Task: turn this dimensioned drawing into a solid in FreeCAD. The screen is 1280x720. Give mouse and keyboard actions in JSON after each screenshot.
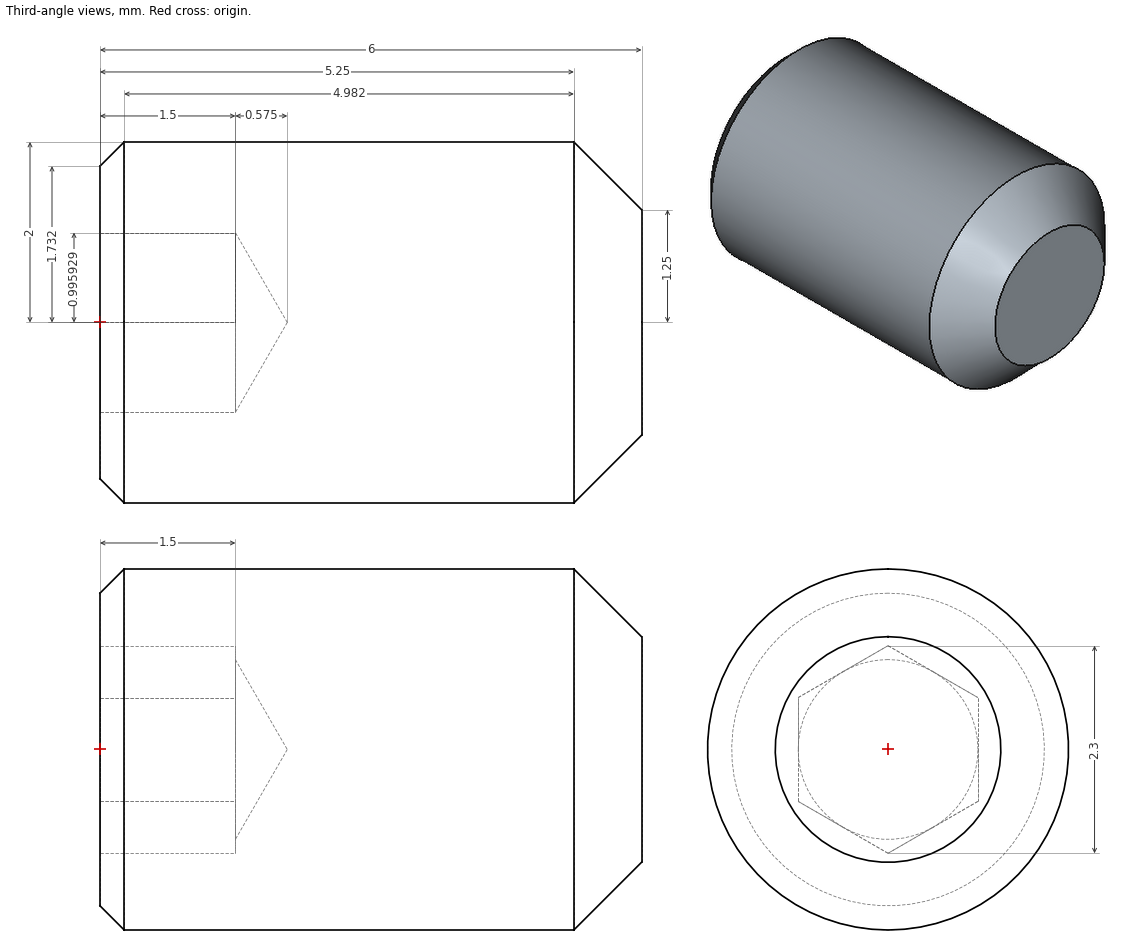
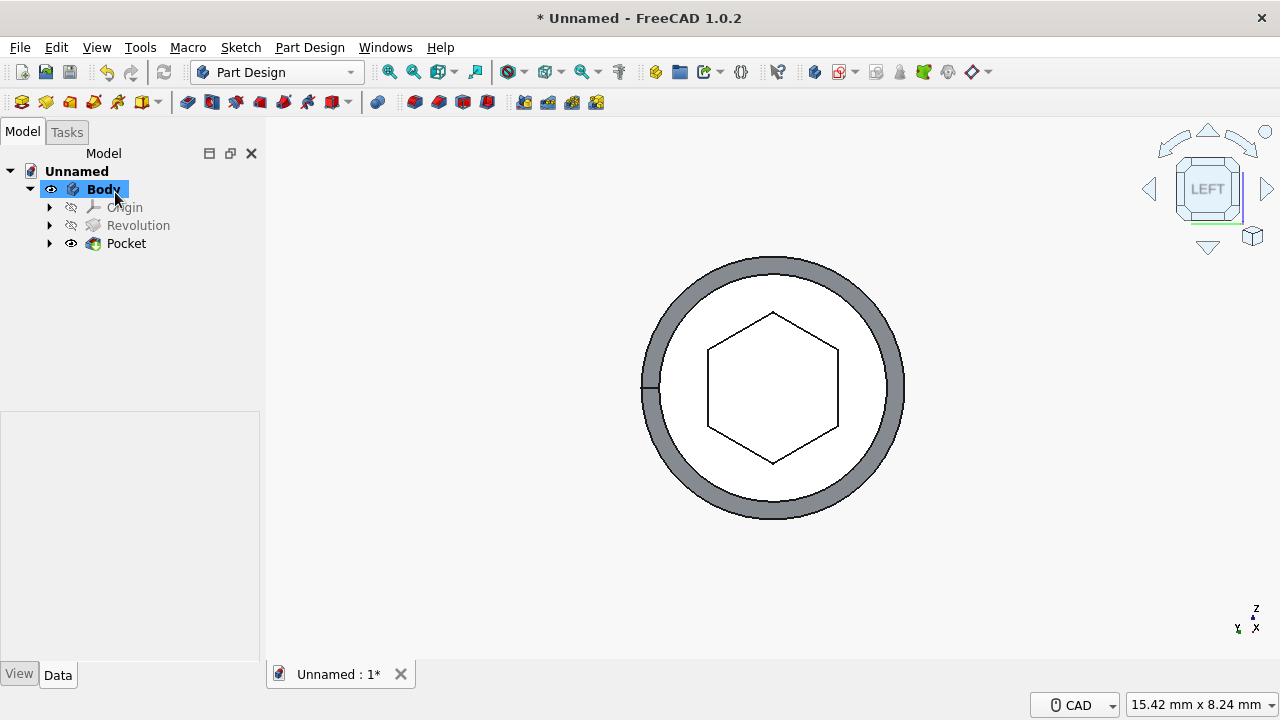
{"action": "left_click", "coordinate": [840, 72]}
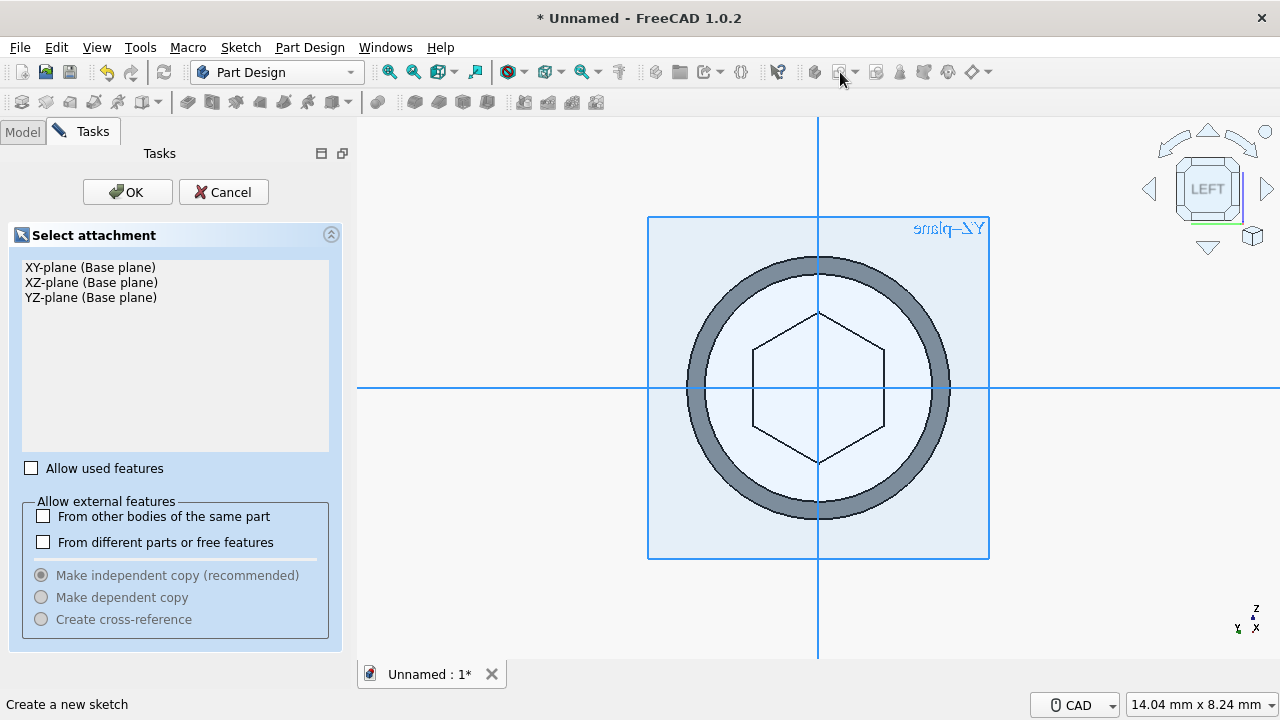
{"action": "left_click", "coordinate": [82, 268]}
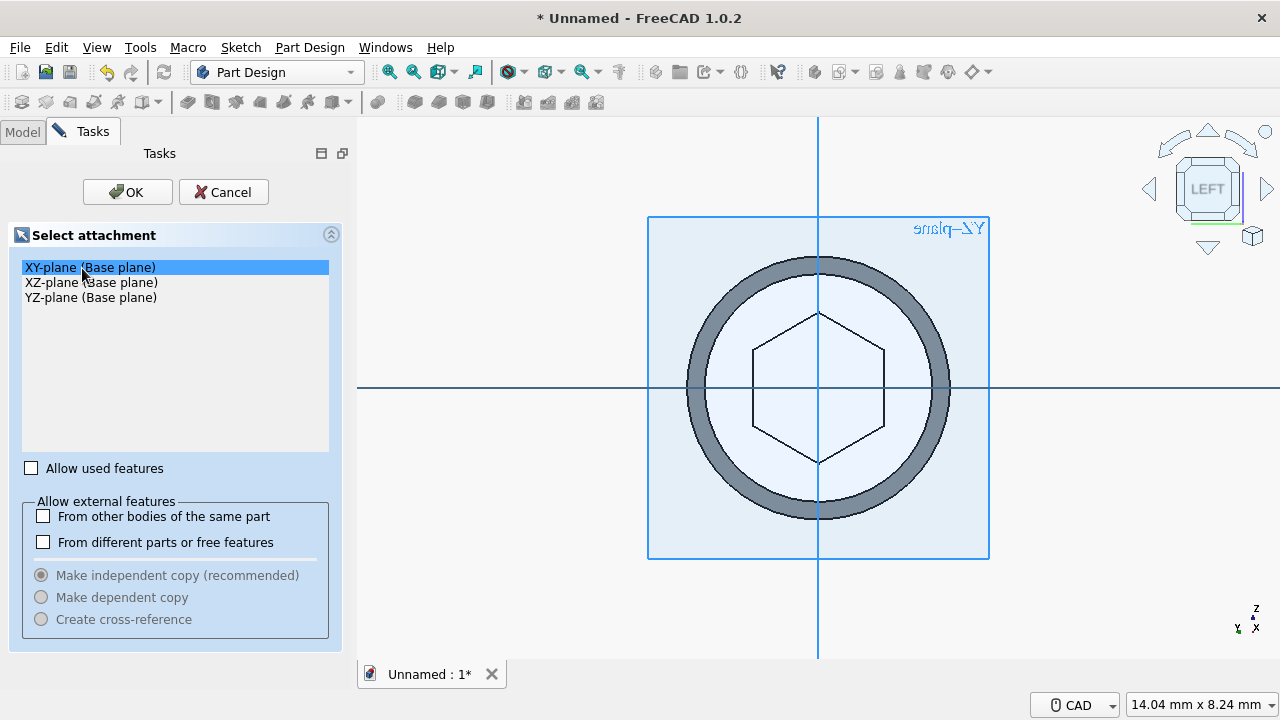
{"action": "left_click", "coordinate": [128, 192]}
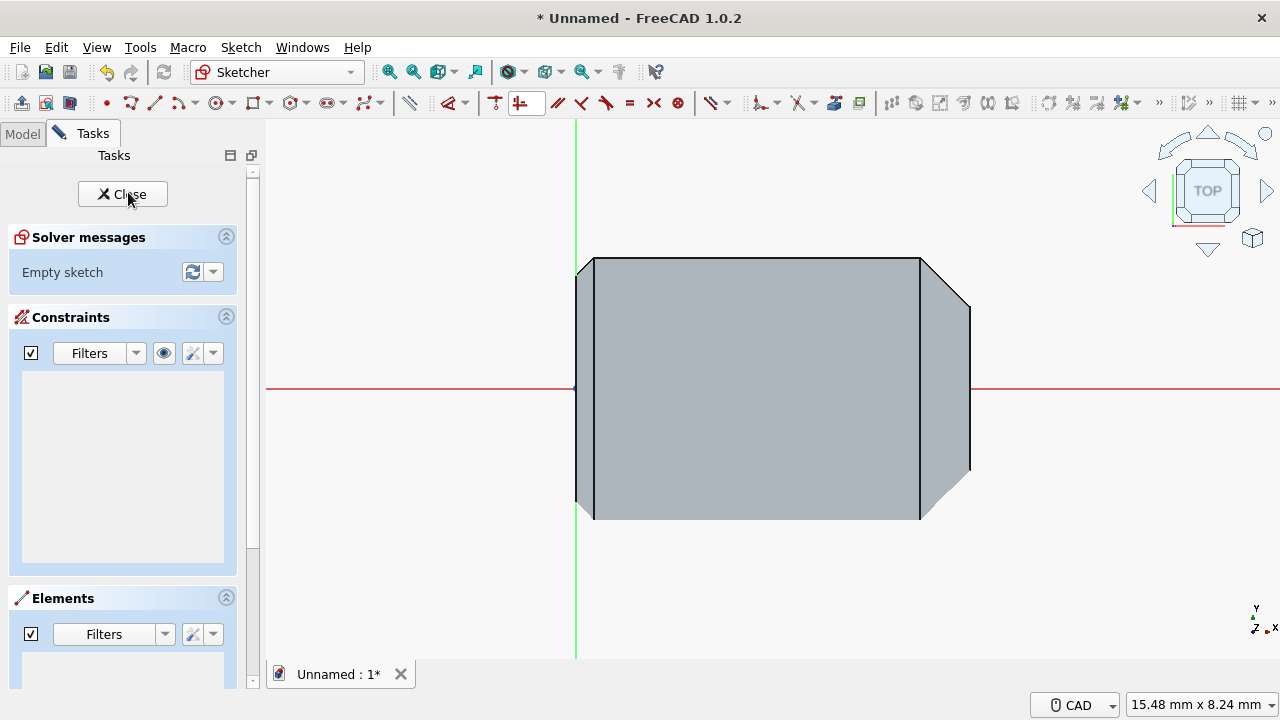
{"action": "left_click", "coordinate": [70, 104]}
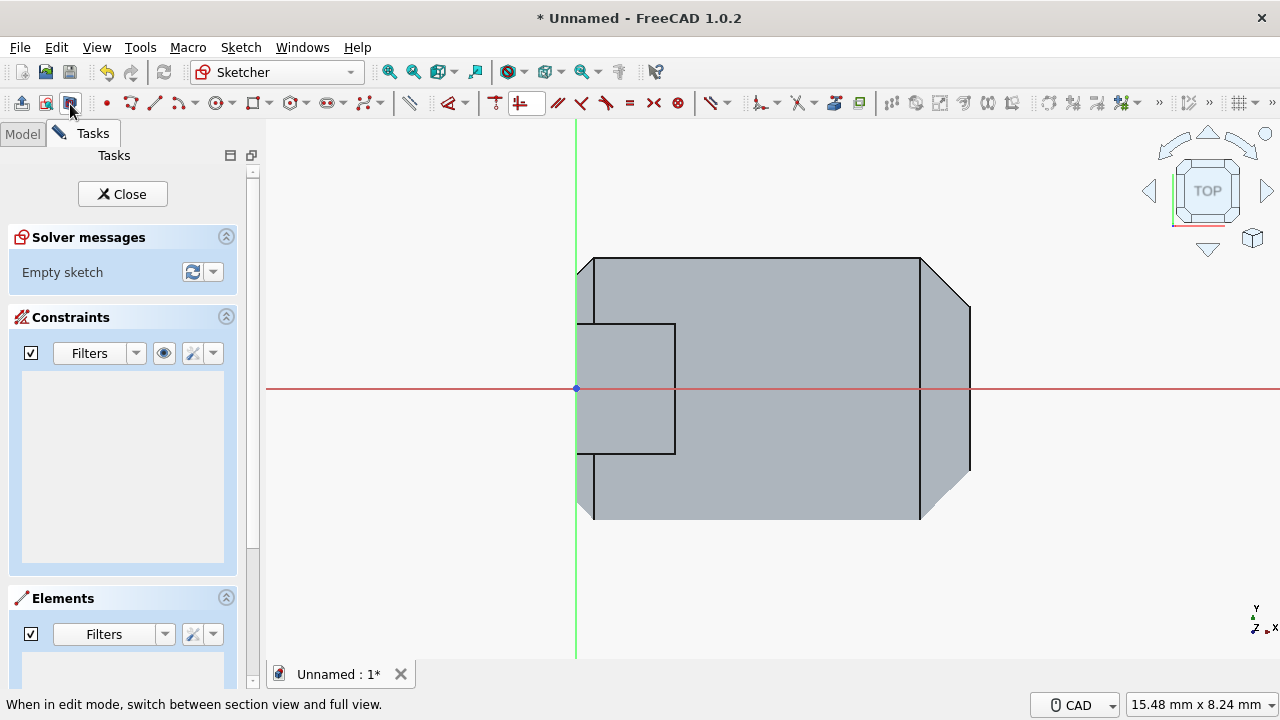
{"action": "scroll", "coordinate": [625, 346], "scroll_direction": "up", "scroll_amount": 7}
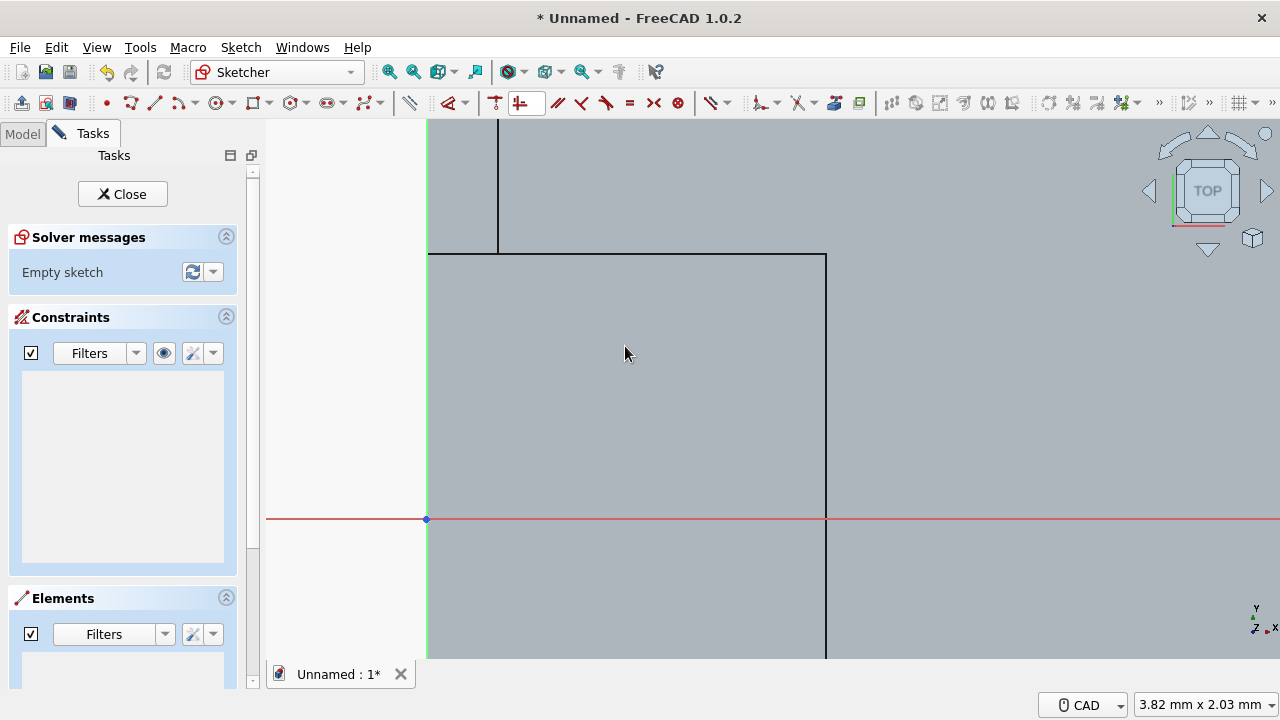
{"action": "left_click", "coordinate": [132, 104]}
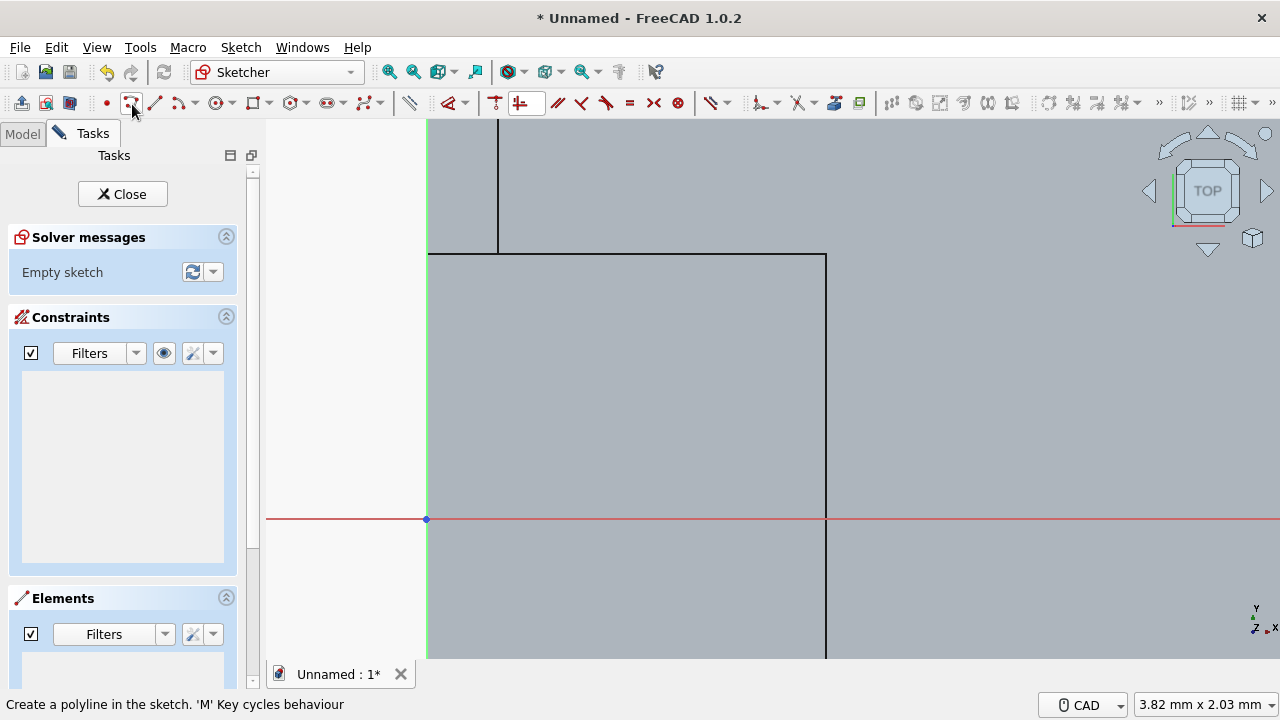
{"action": "left_click", "coordinate": [826, 519]}
{"action": "left_click", "coordinate": [978, 510]}
{"action": "left_click", "coordinate": [826, 254]}
{"action": "left_click", "coordinate": [826, 519]}
{"action": "key", "text": "Escape"}
{"action": "key", "text": "Escape"}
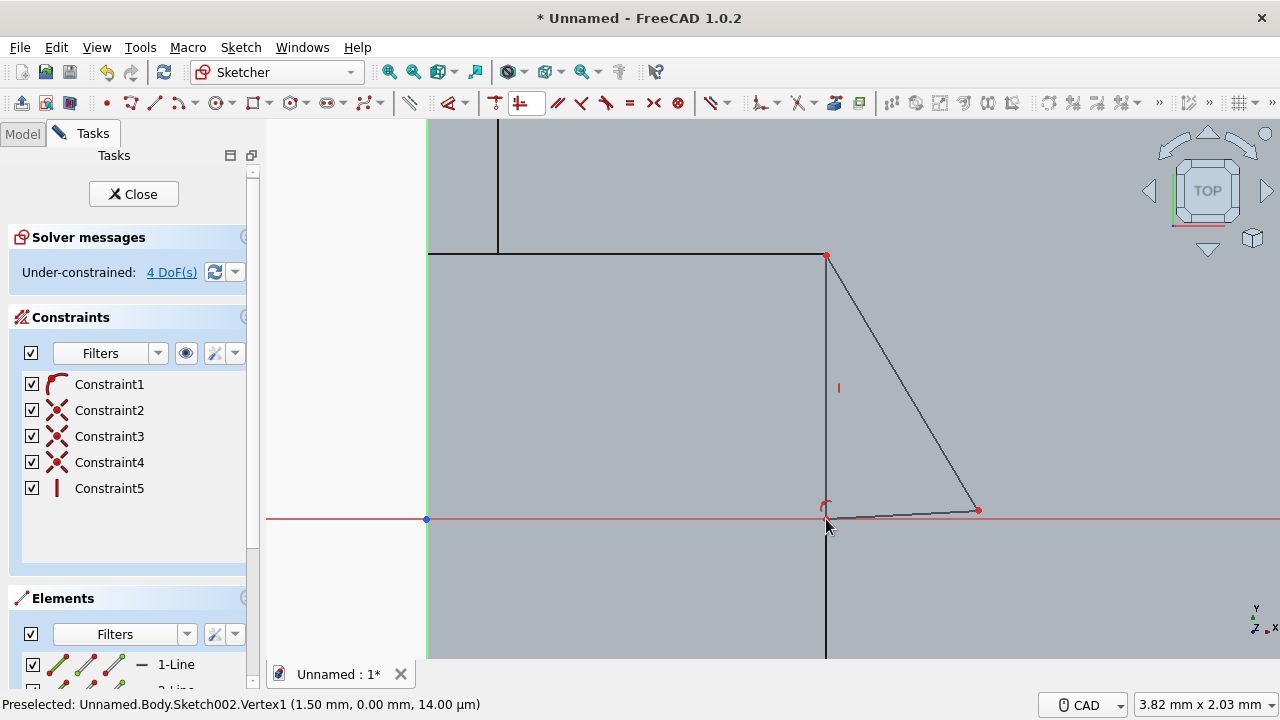
{"action": "left_click", "coordinate": [872, 517]}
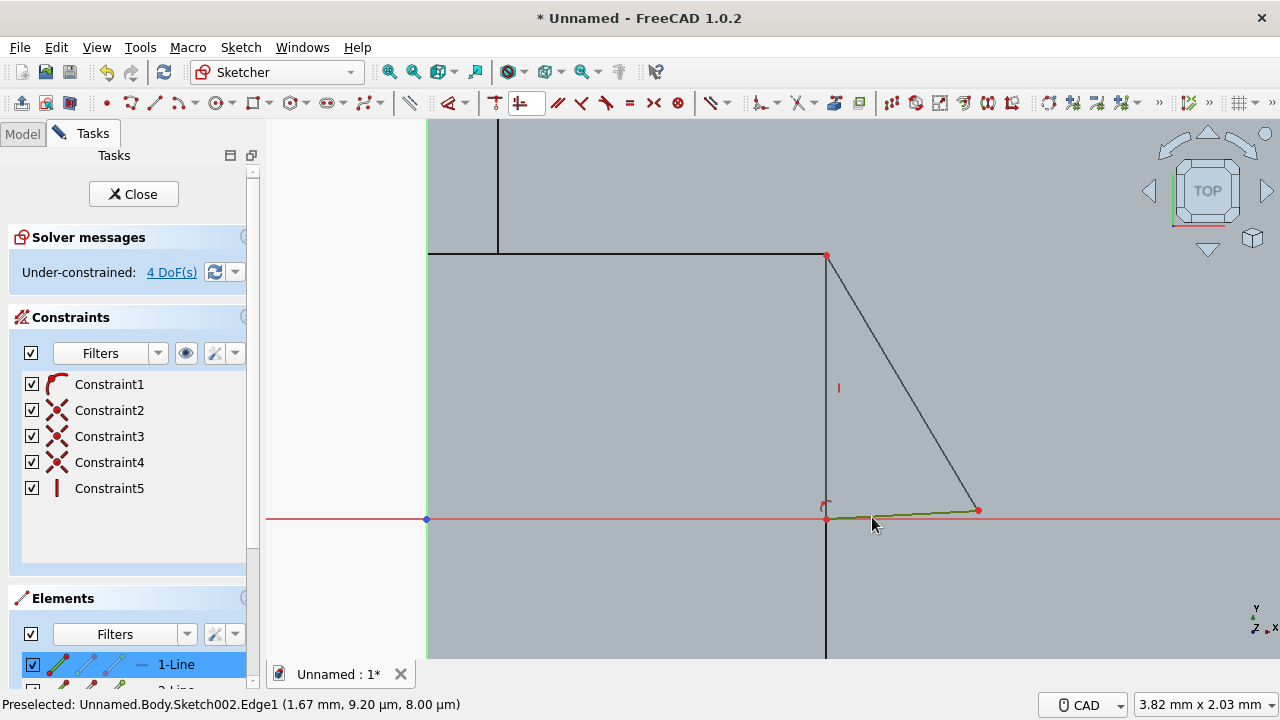
{"action": "left_click", "coordinate": [540, 104]}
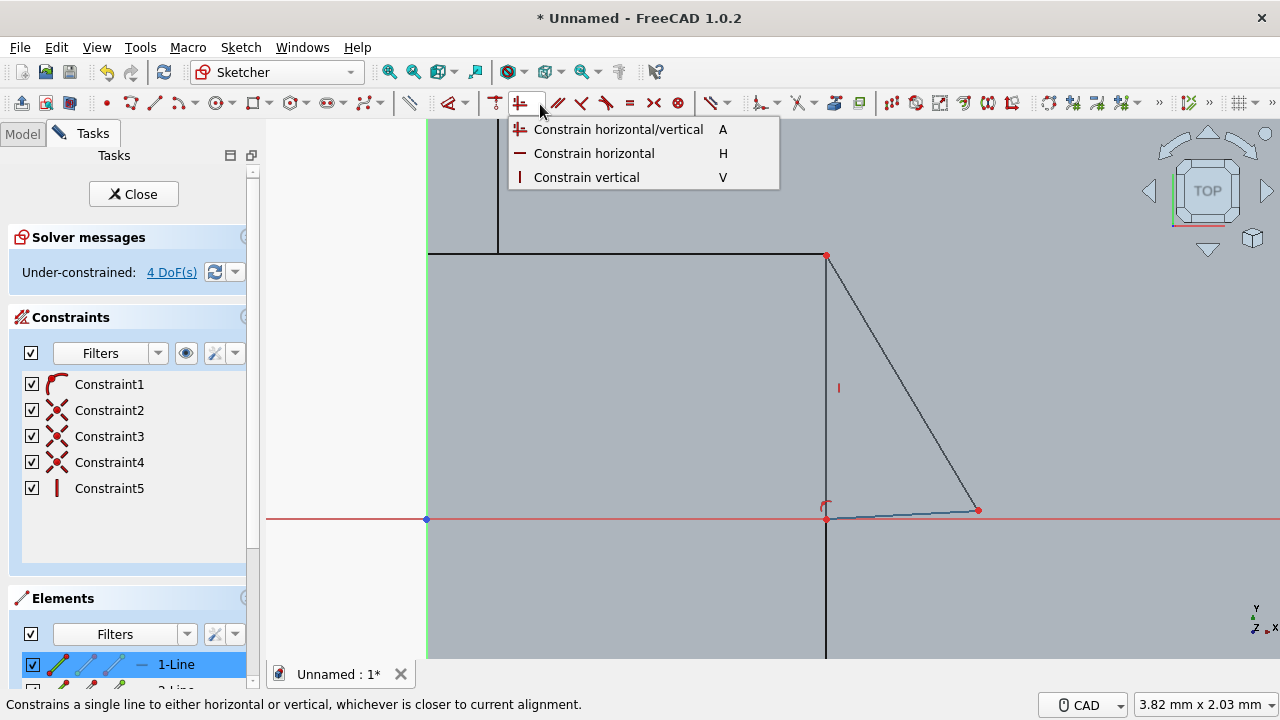
{"action": "left_click", "coordinate": [644, 153]}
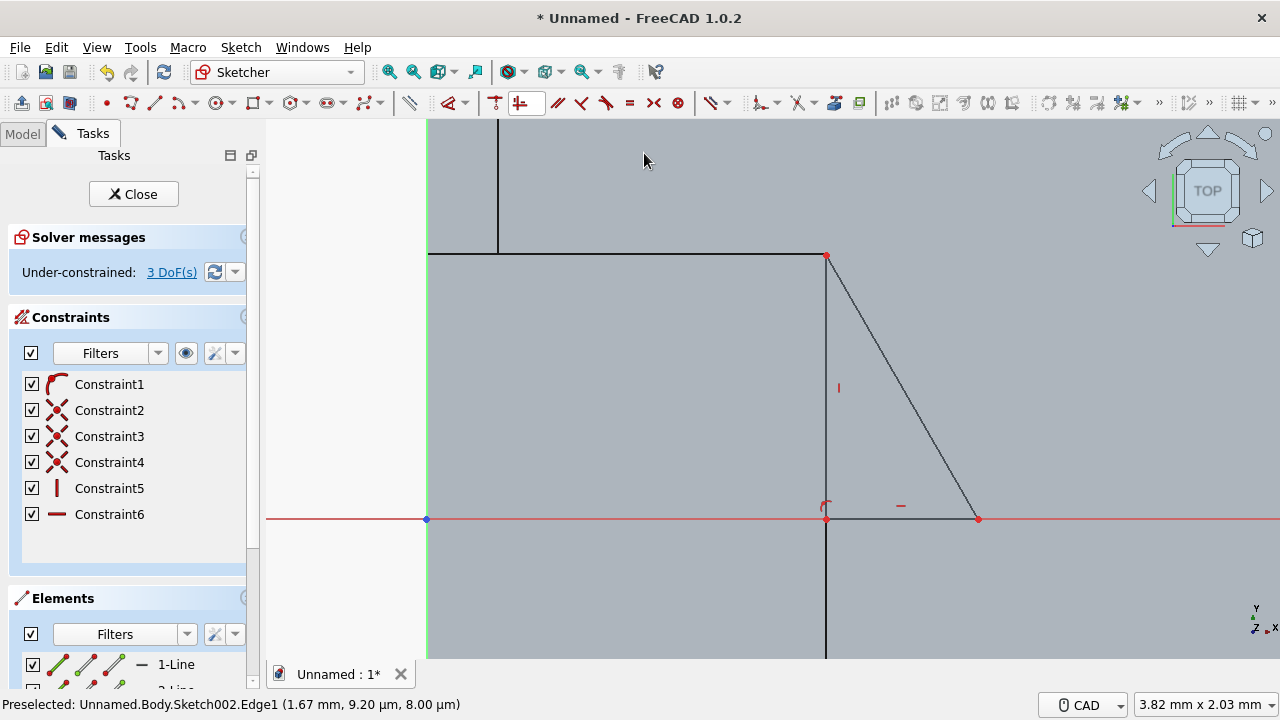
{"action": "left_click", "coordinate": [448, 104]}